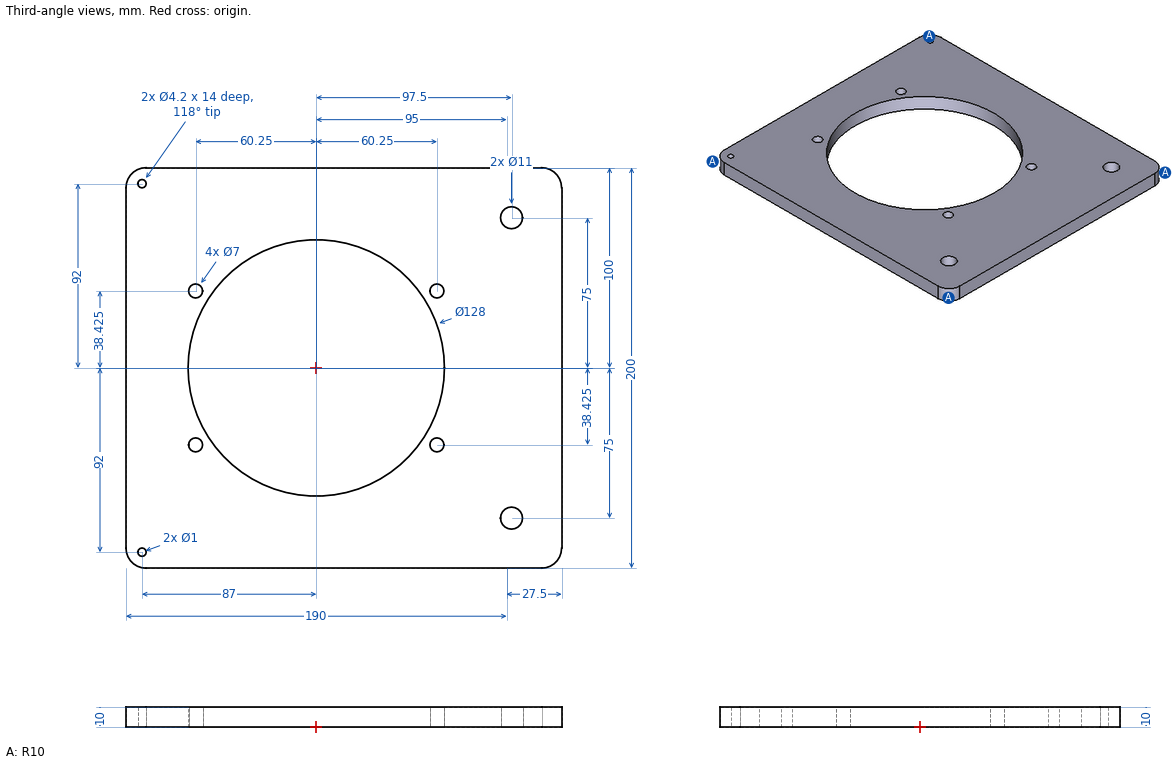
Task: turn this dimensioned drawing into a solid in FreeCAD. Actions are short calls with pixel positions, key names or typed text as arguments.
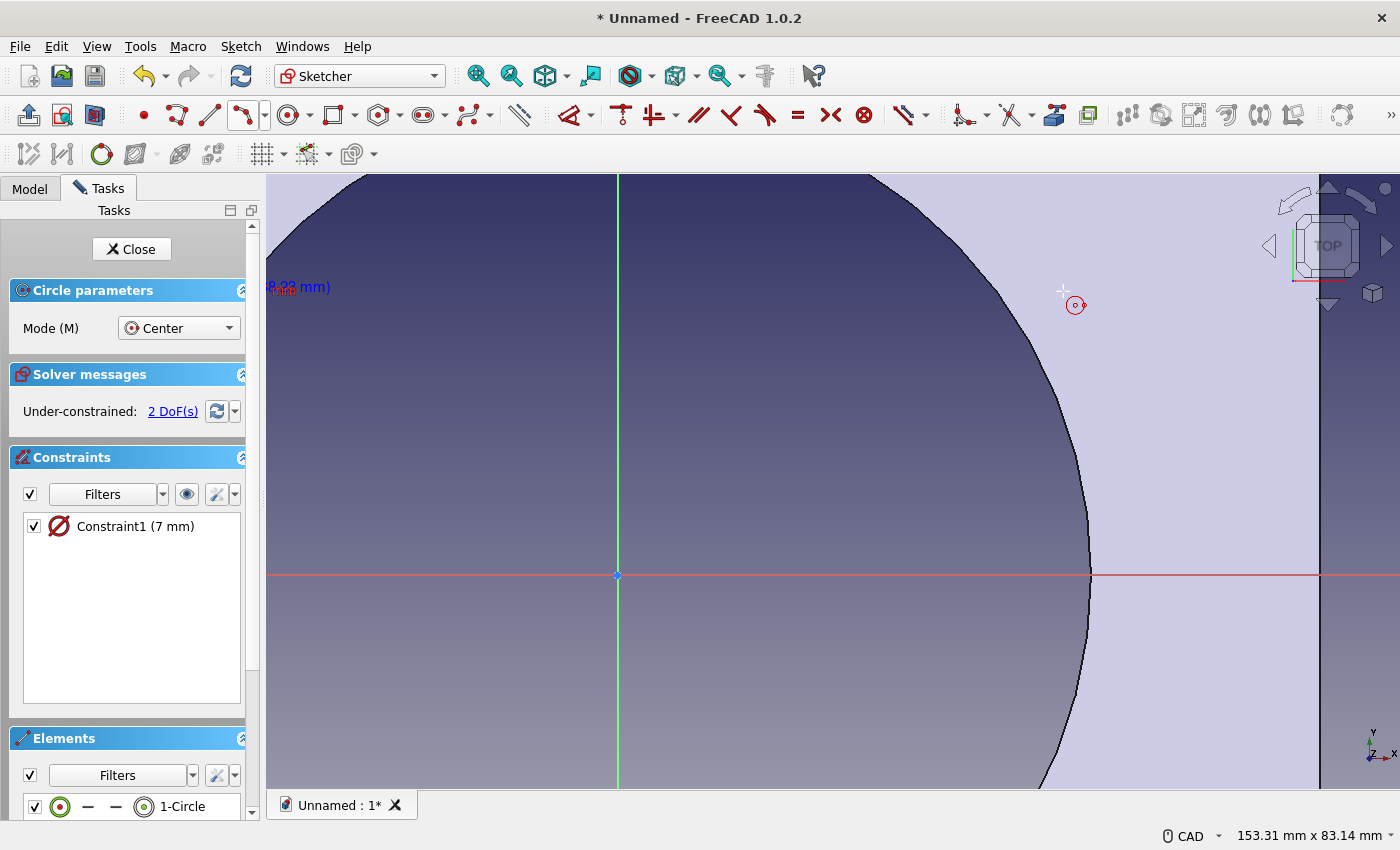
click(1063, 291)
move(1082, 273)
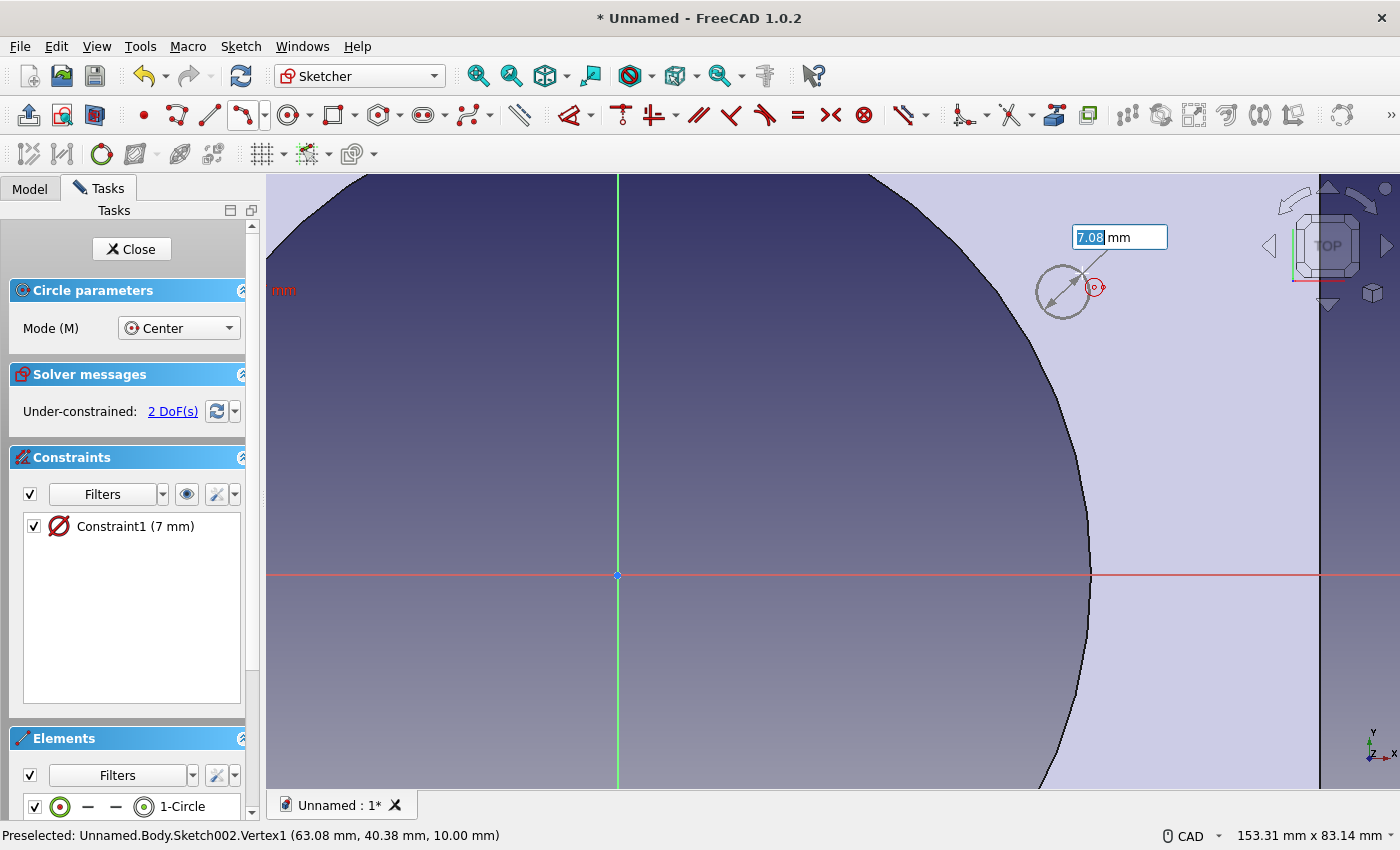
text(7)
key(Return)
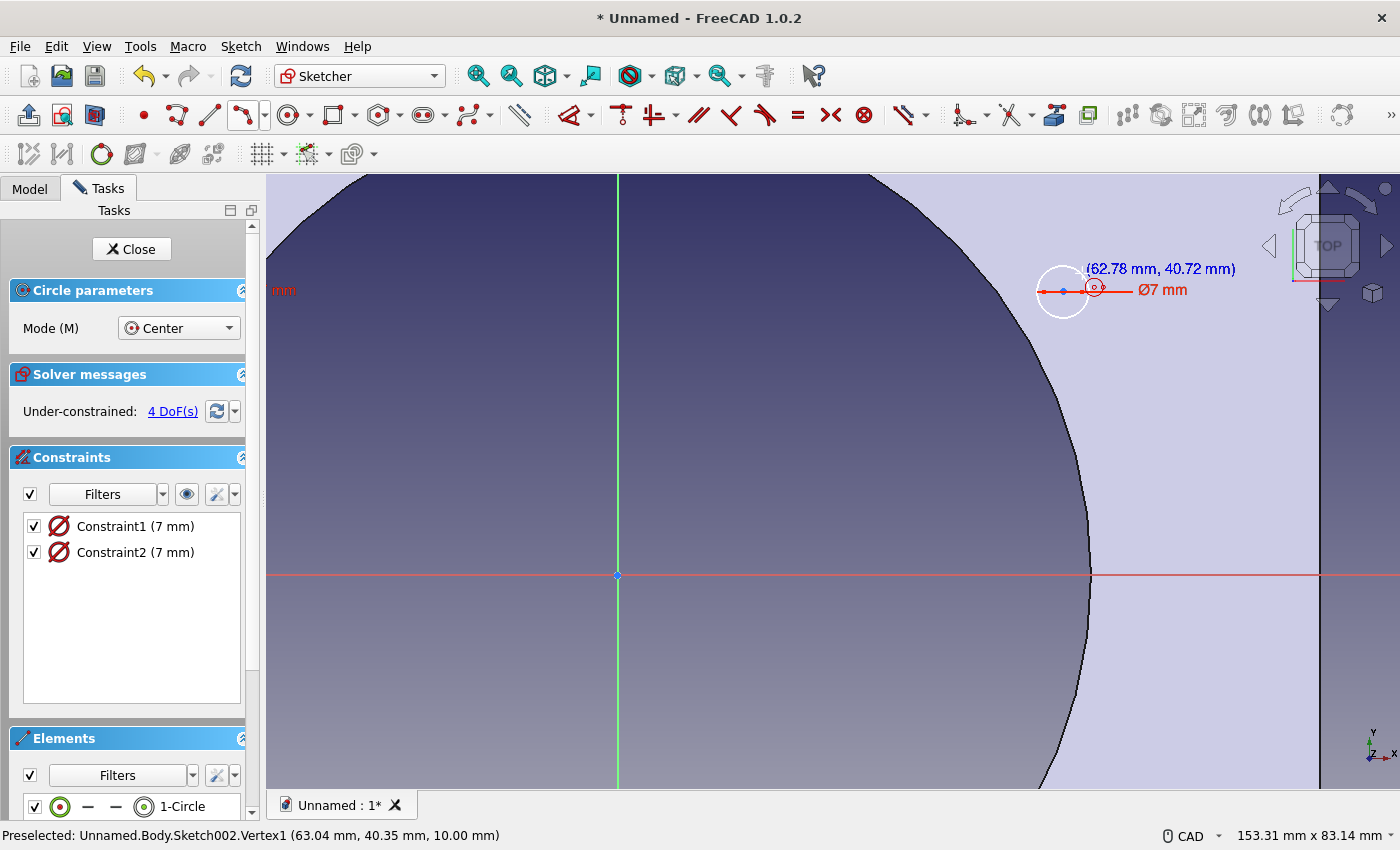
scroll(1063, 291, down, 2)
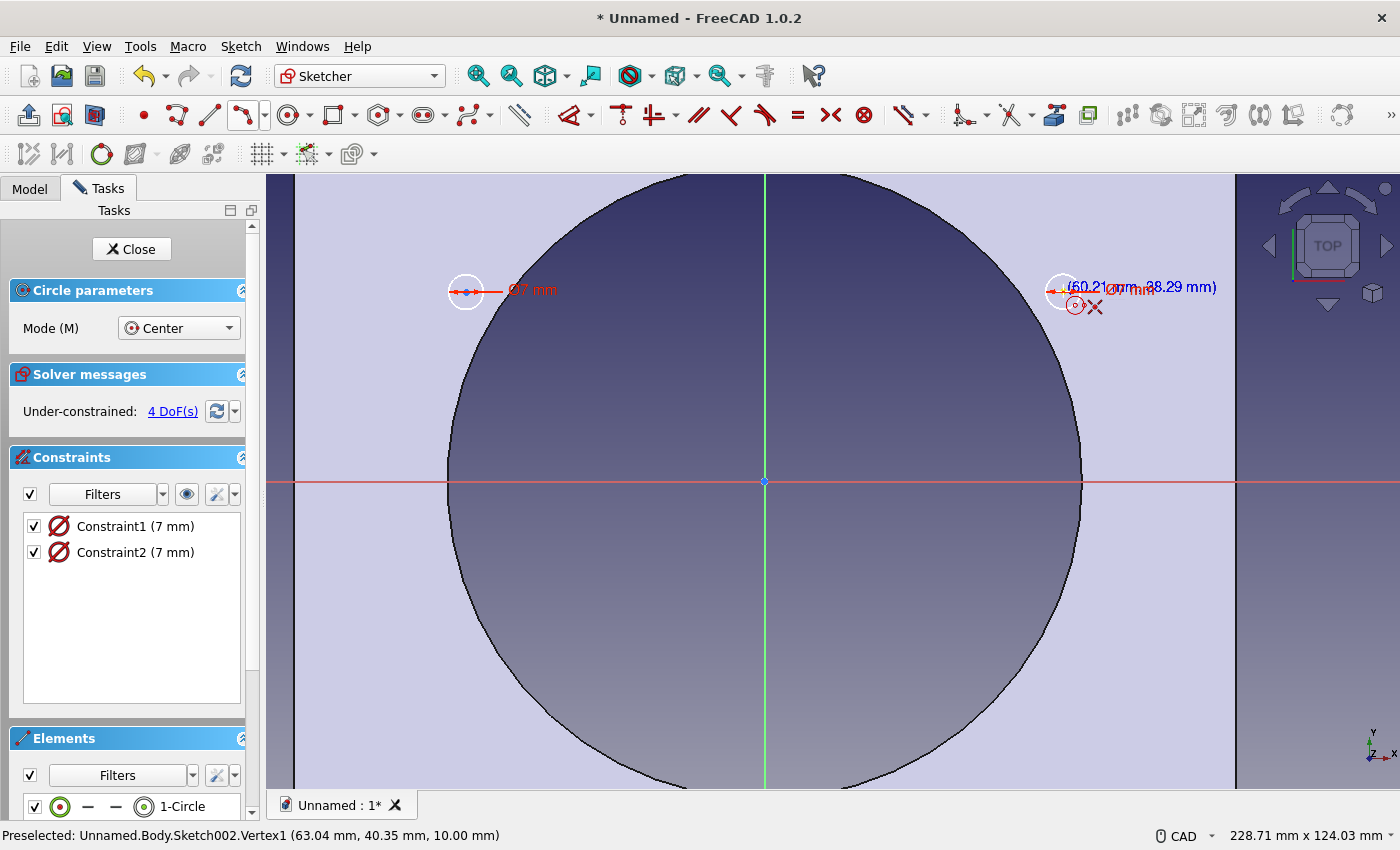
scroll(1063, 672, up, 2)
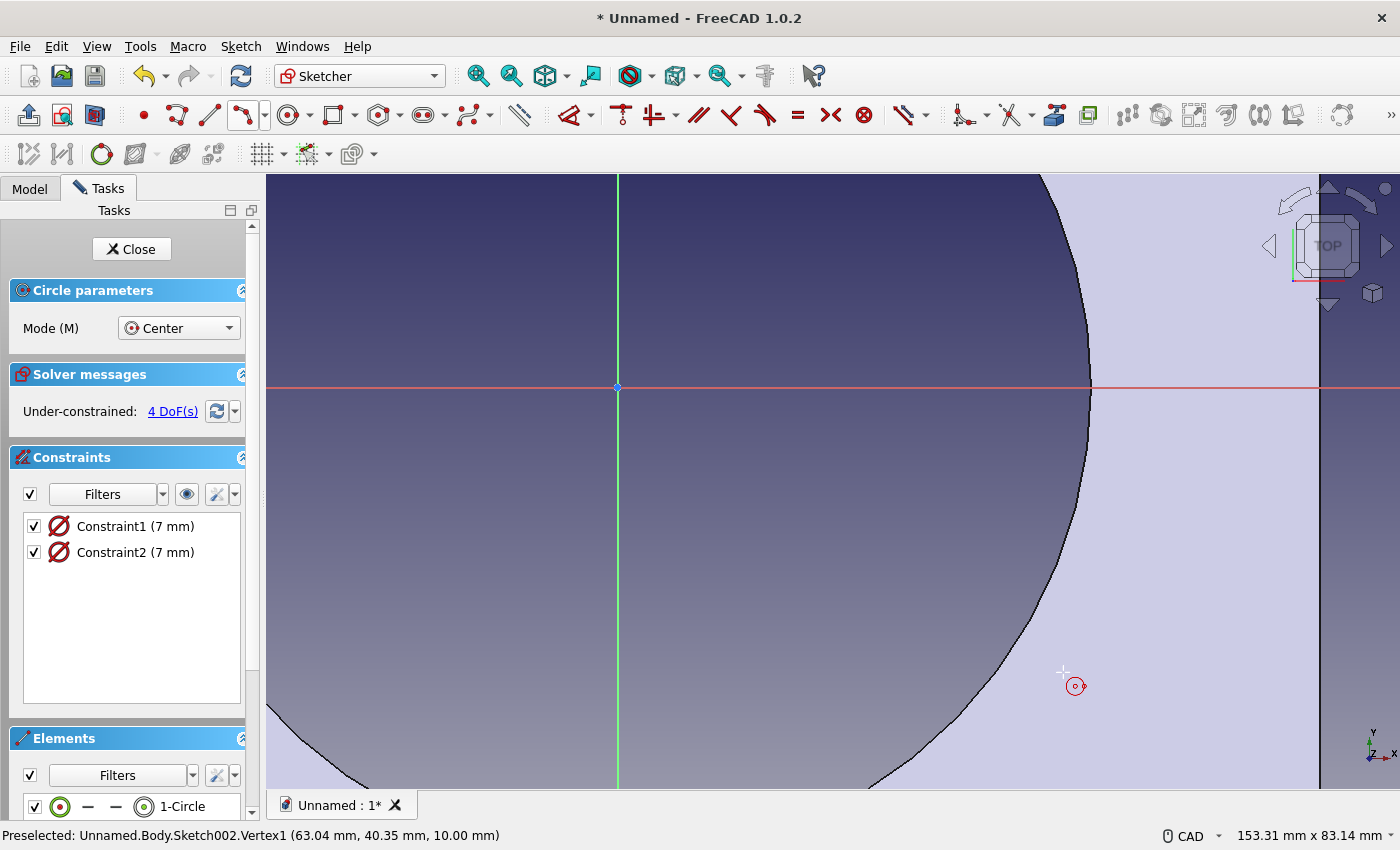
click(1063, 672)
move(1082, 653)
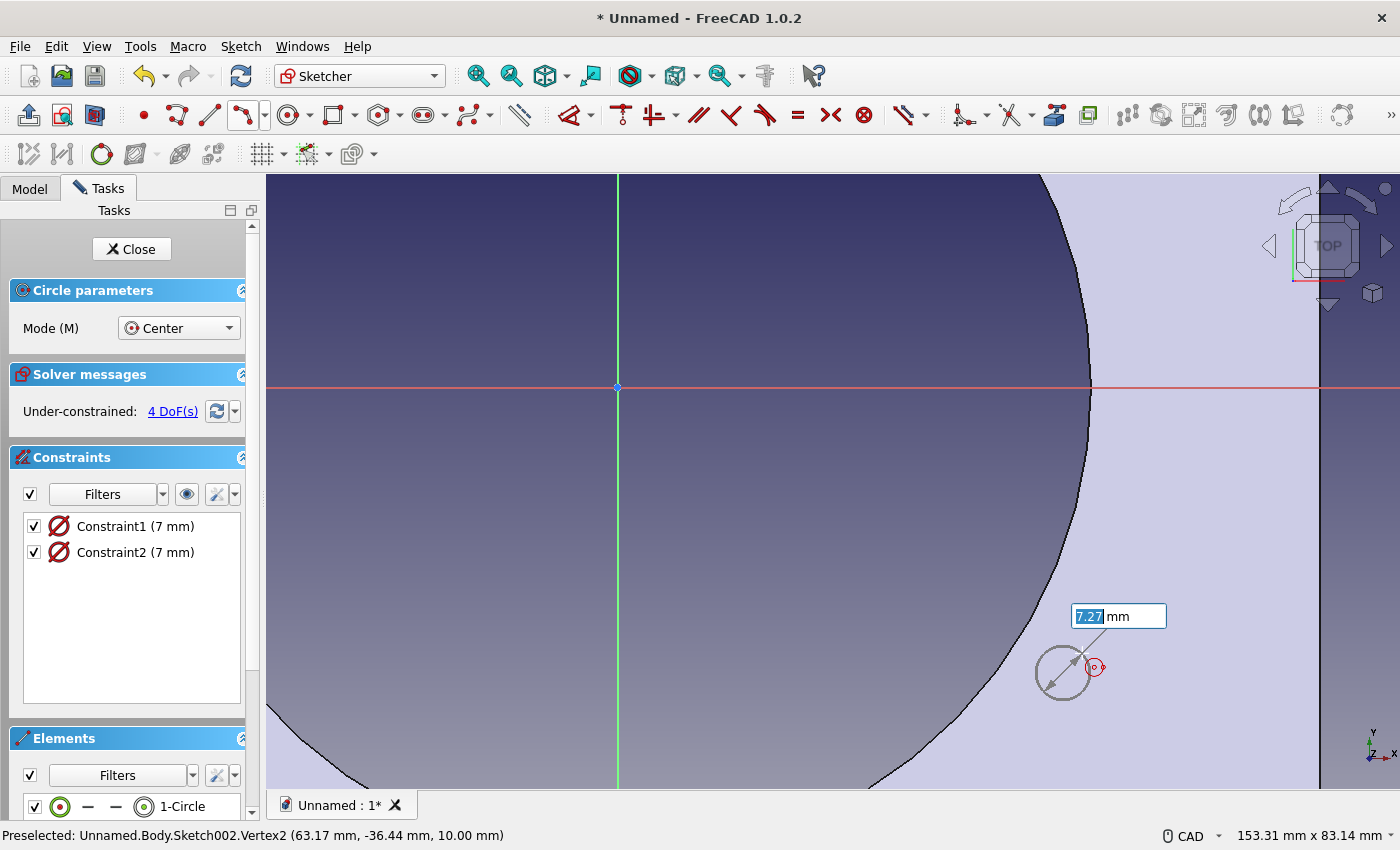
text(7)
key(Return)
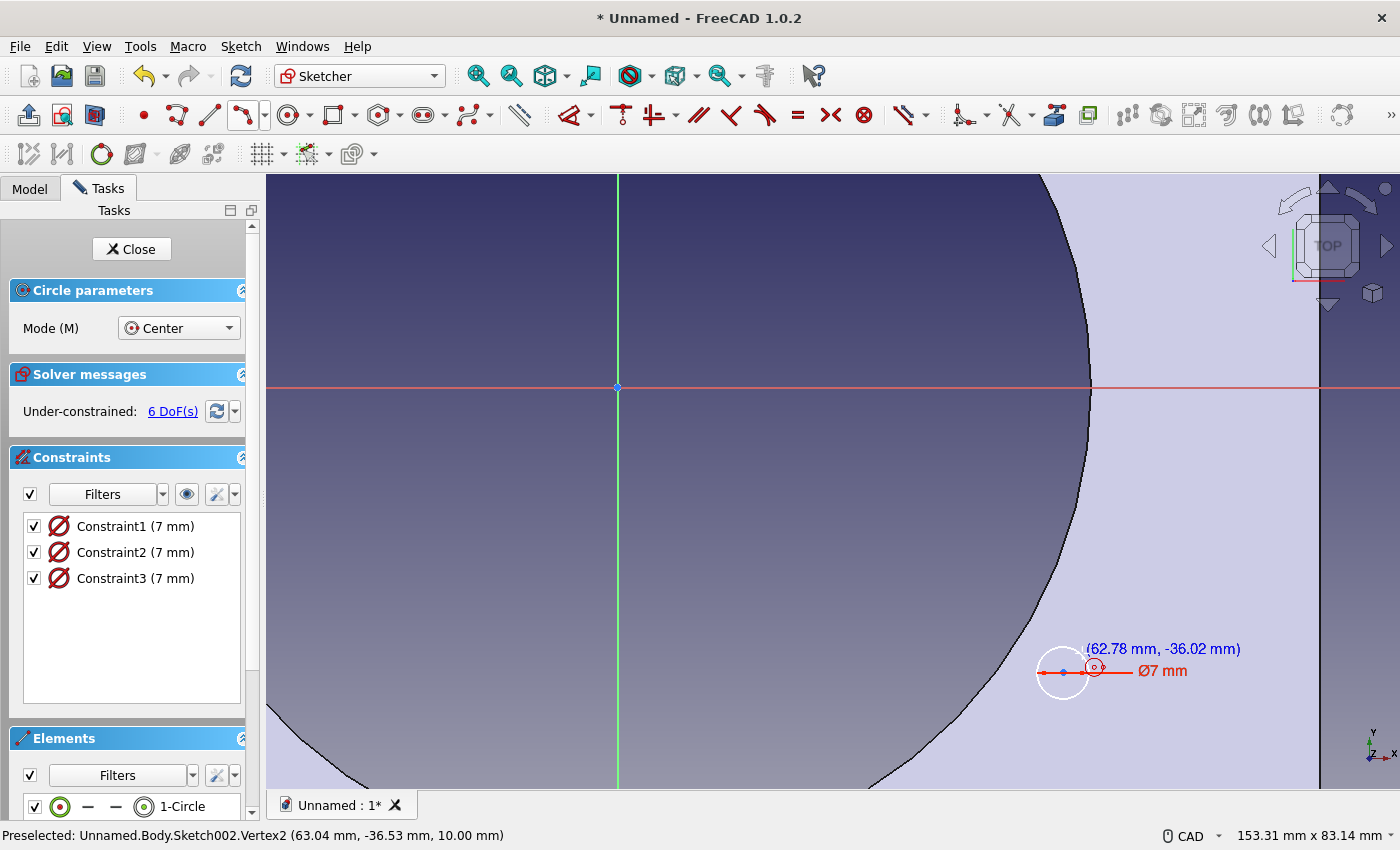
scroll(1063, 673, down, 2)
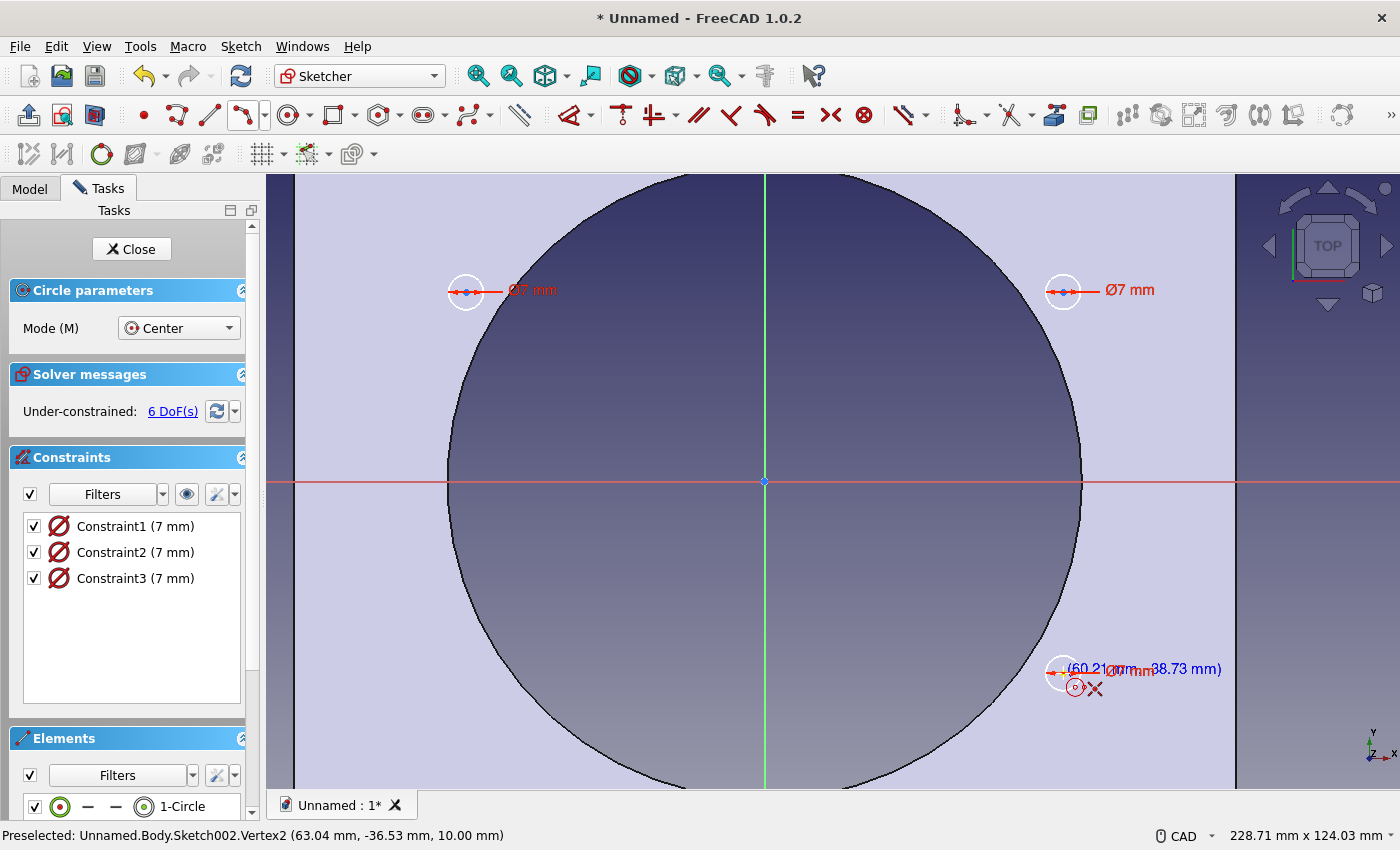
scroll(466, 672, up, 2)